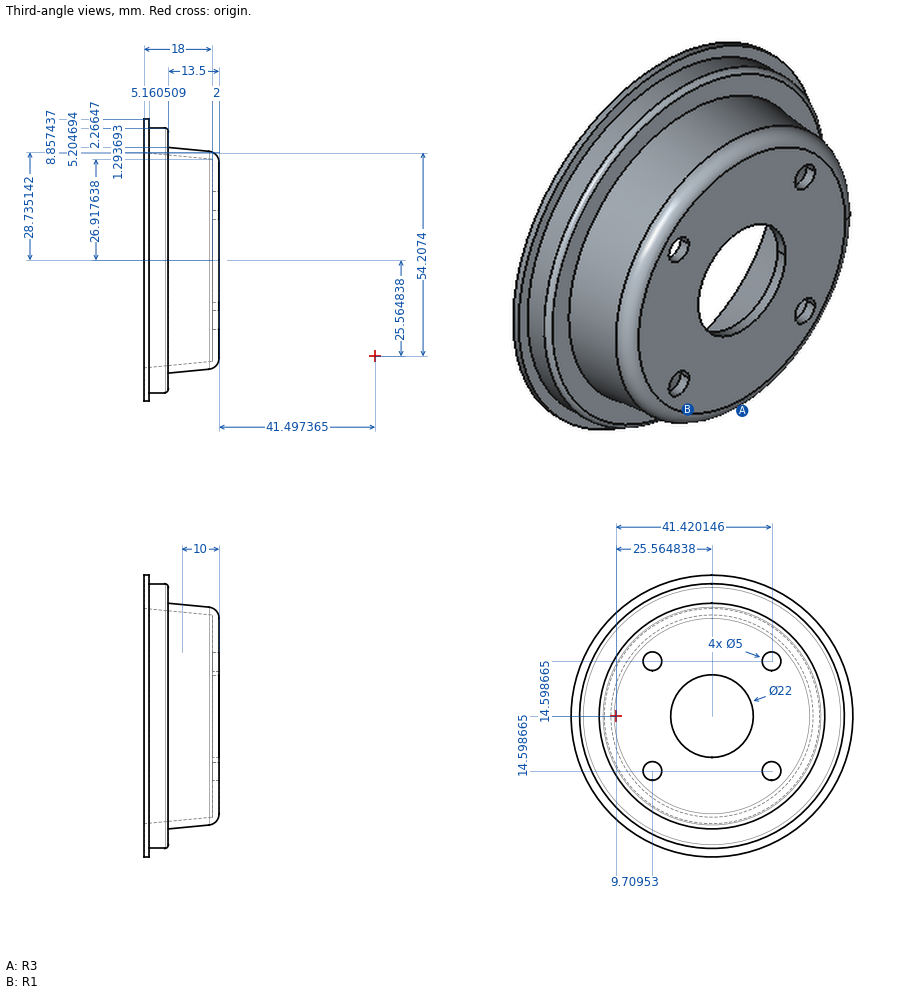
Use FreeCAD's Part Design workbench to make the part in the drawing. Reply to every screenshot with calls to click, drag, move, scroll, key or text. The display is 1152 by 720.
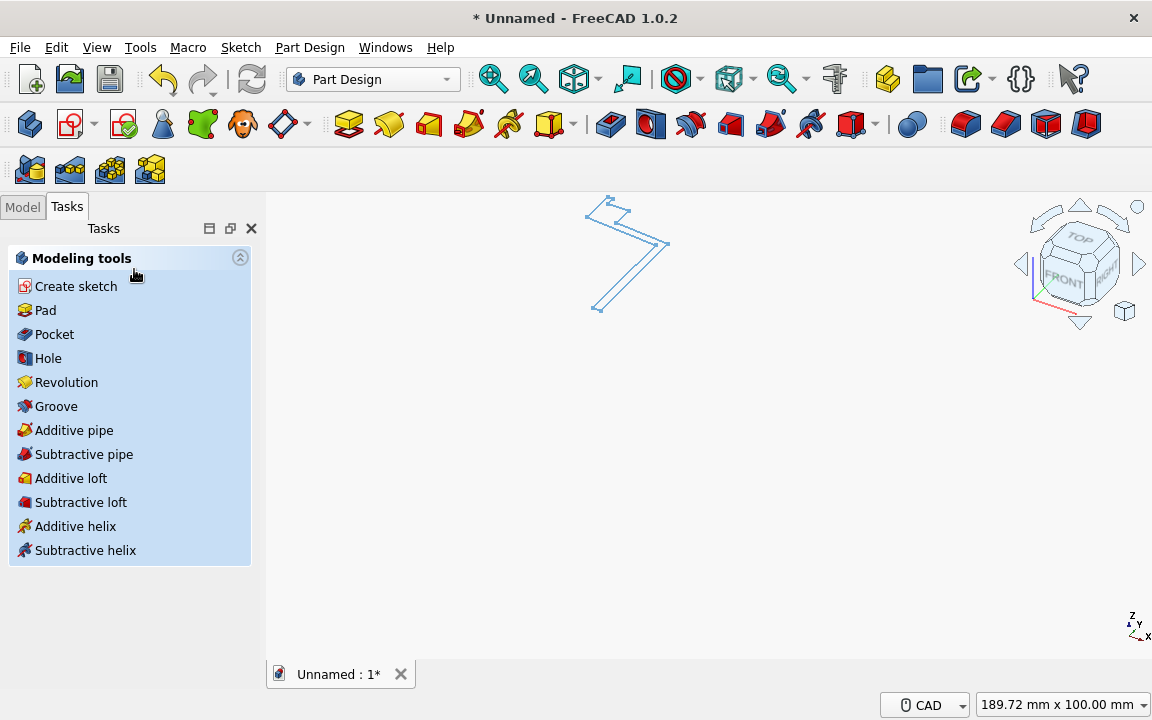
click(390, 124)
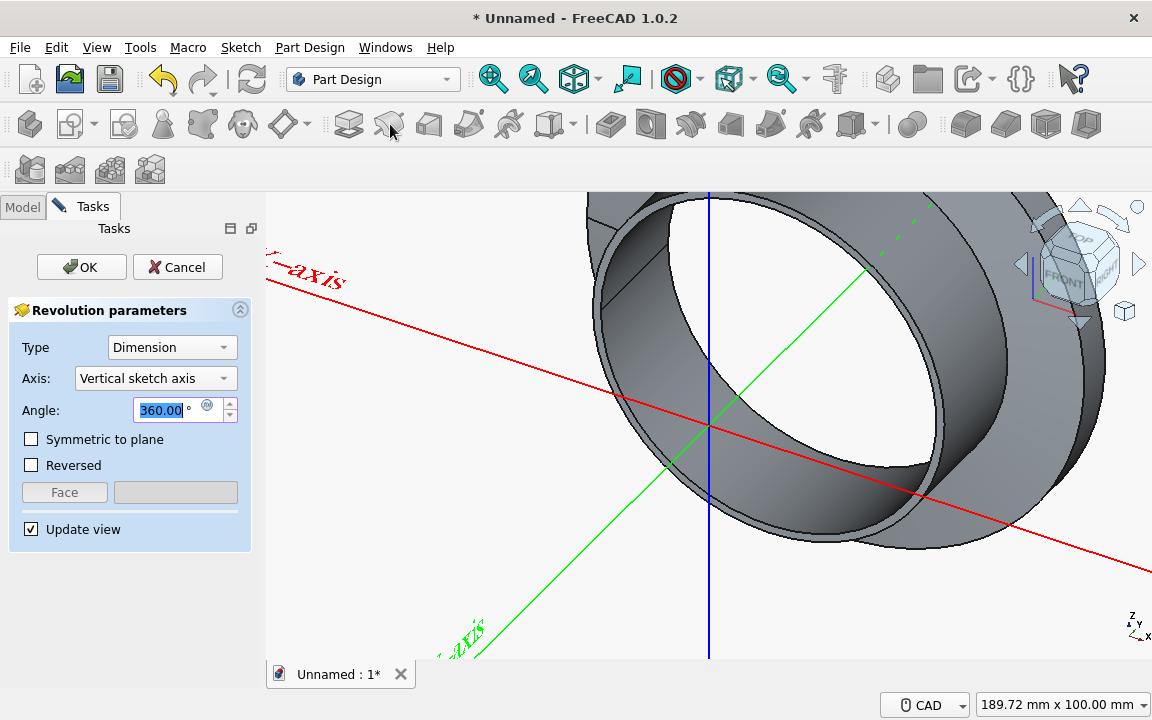
click(156, 378)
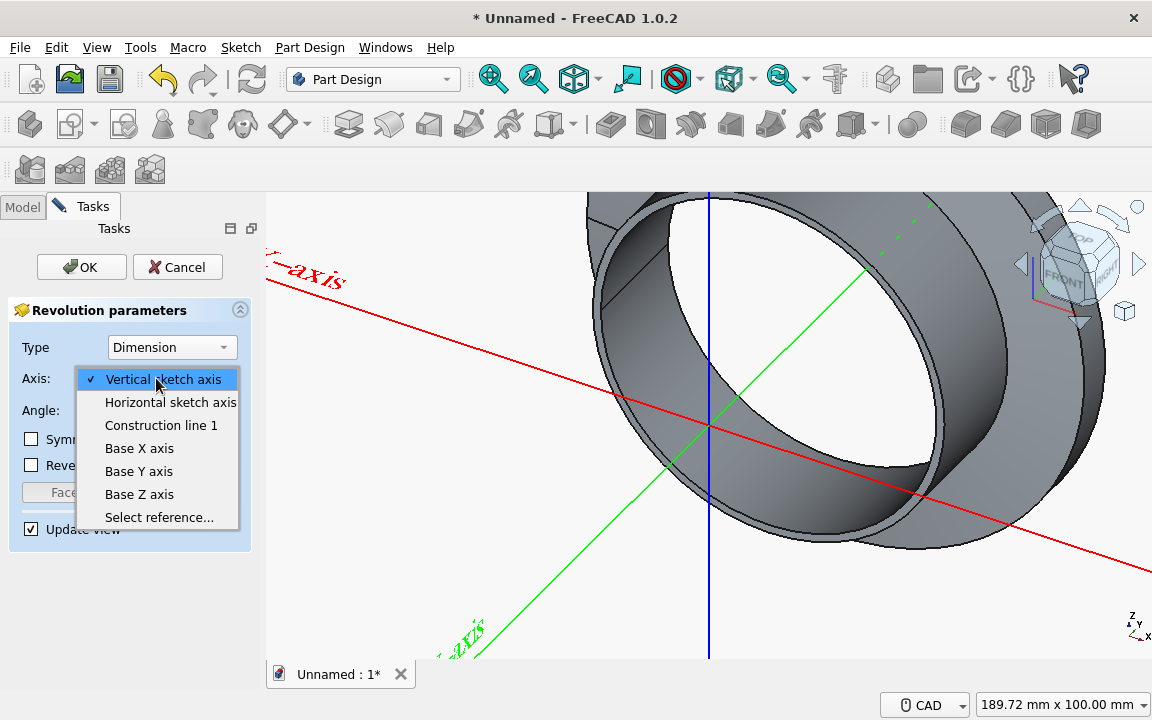
click(156, 426)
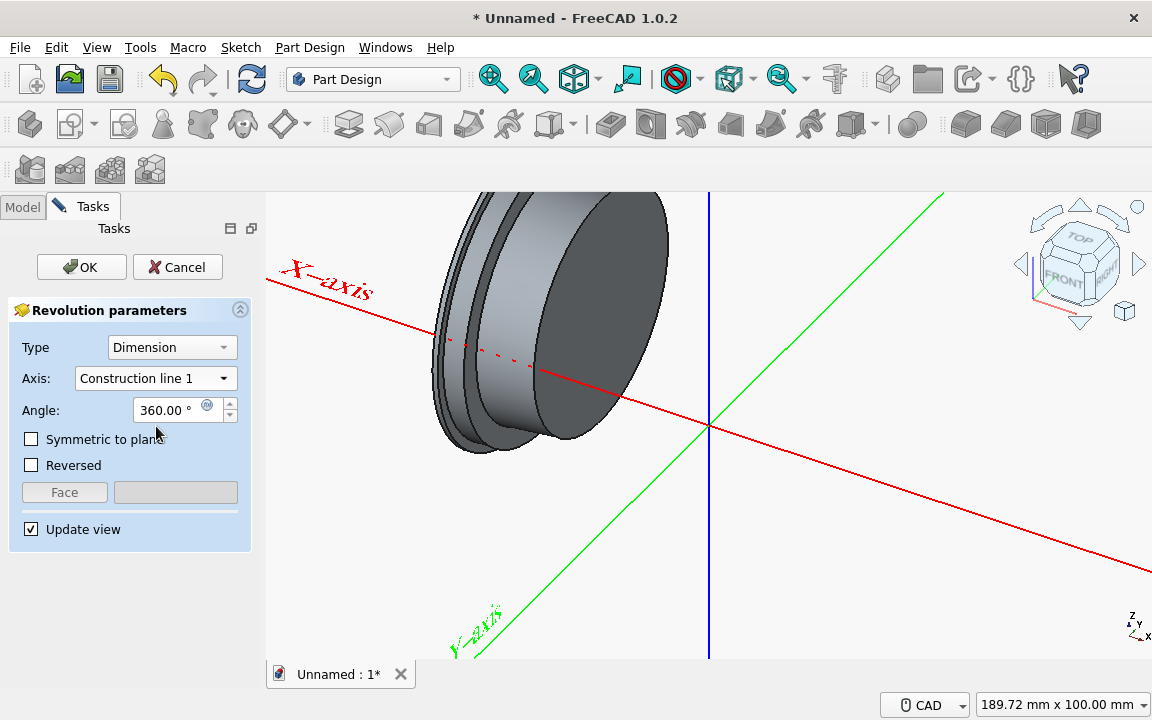
click(82, 267)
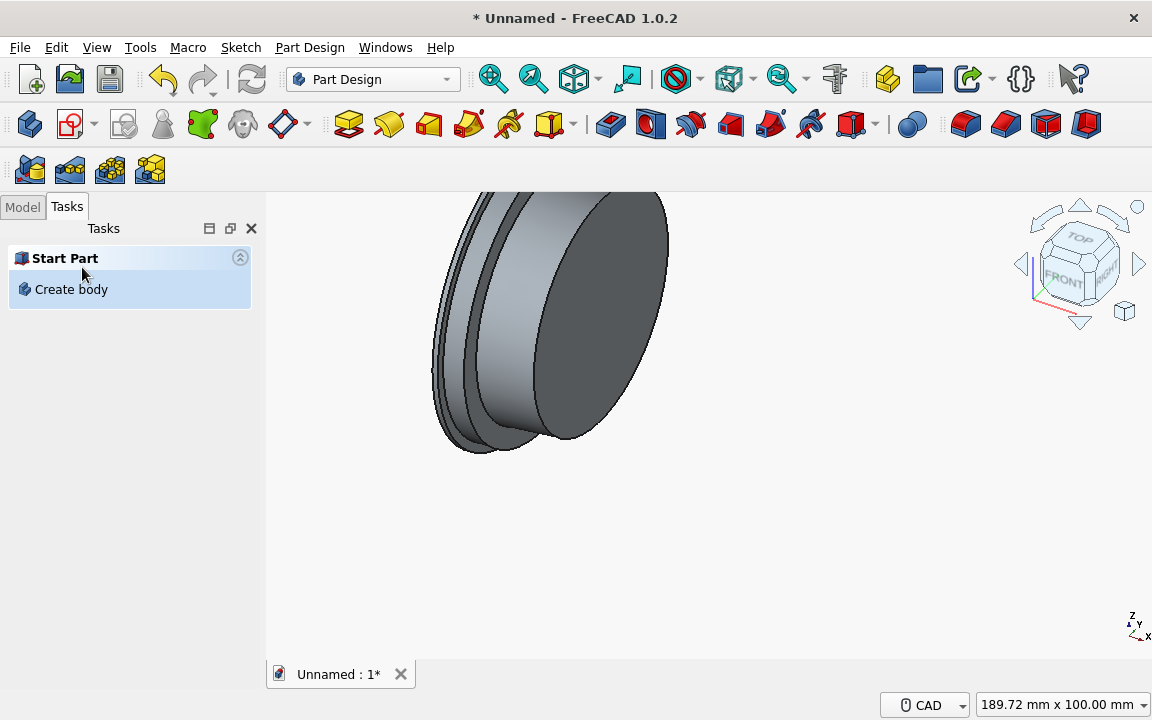
key(v)
key(f)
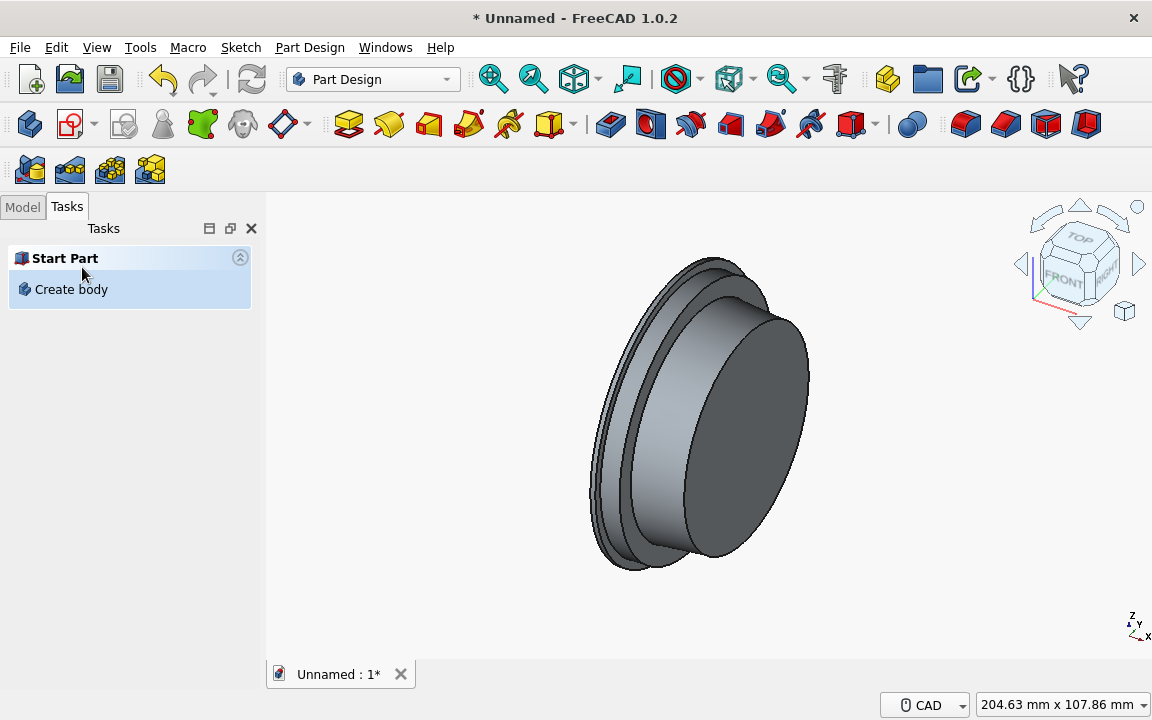
click(746, 437)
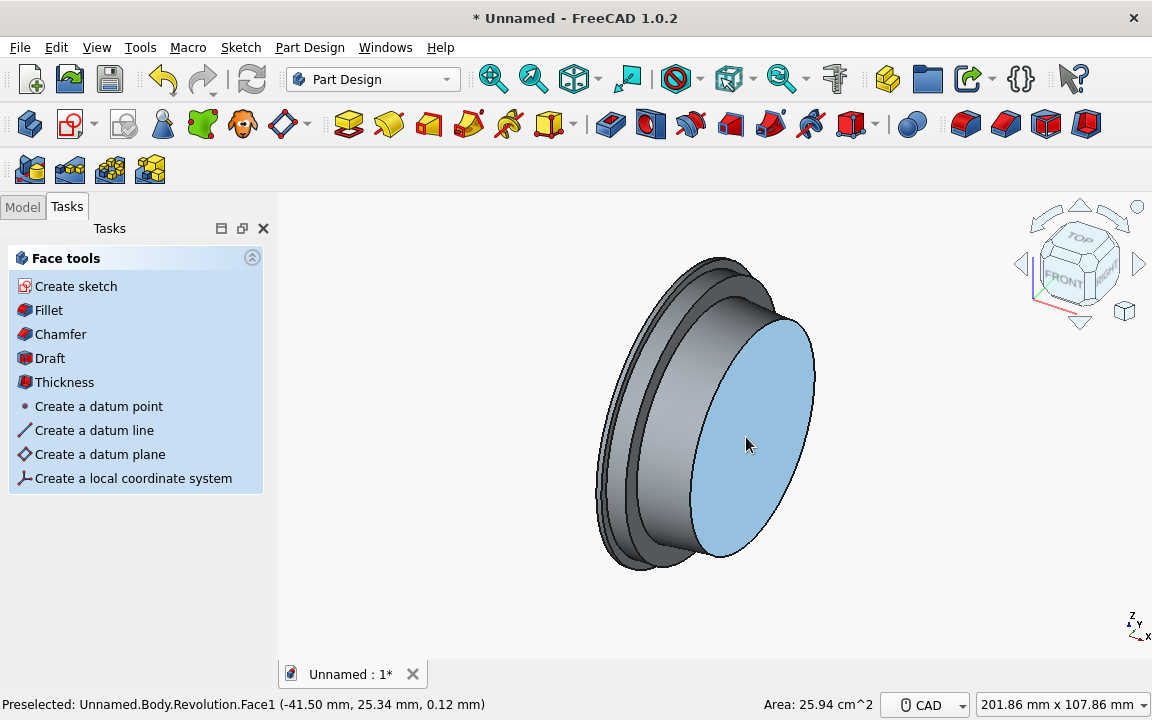
click(70, 124)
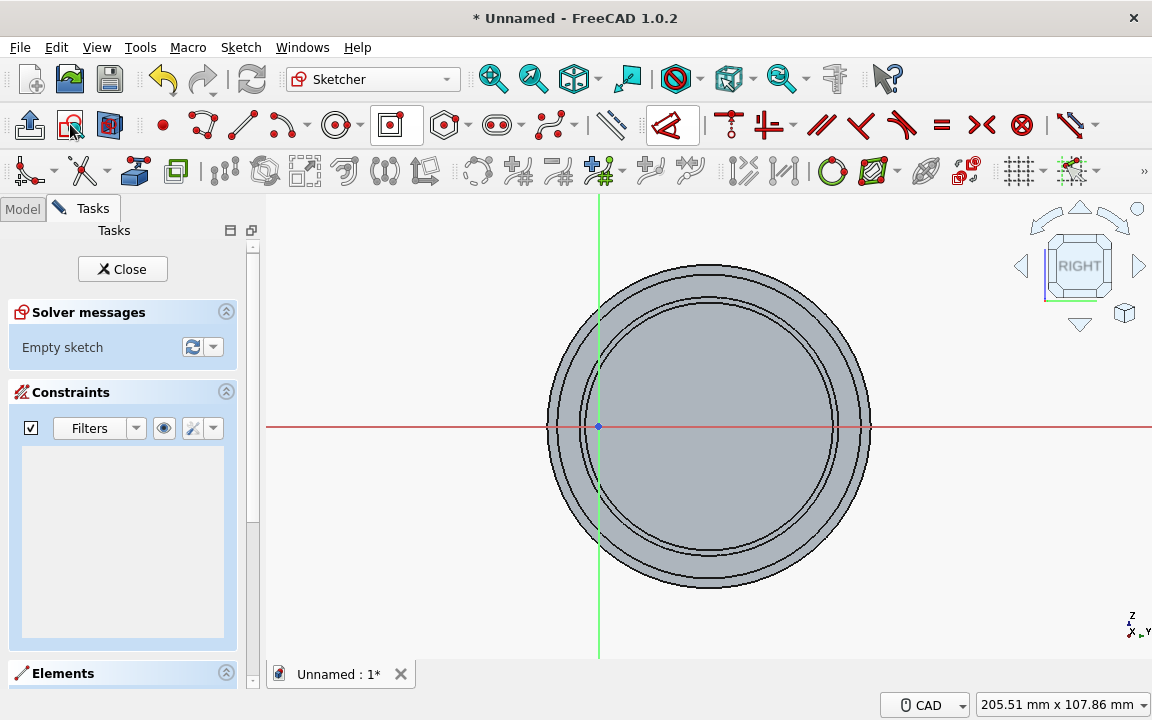
scroll(758, 426, up, 3)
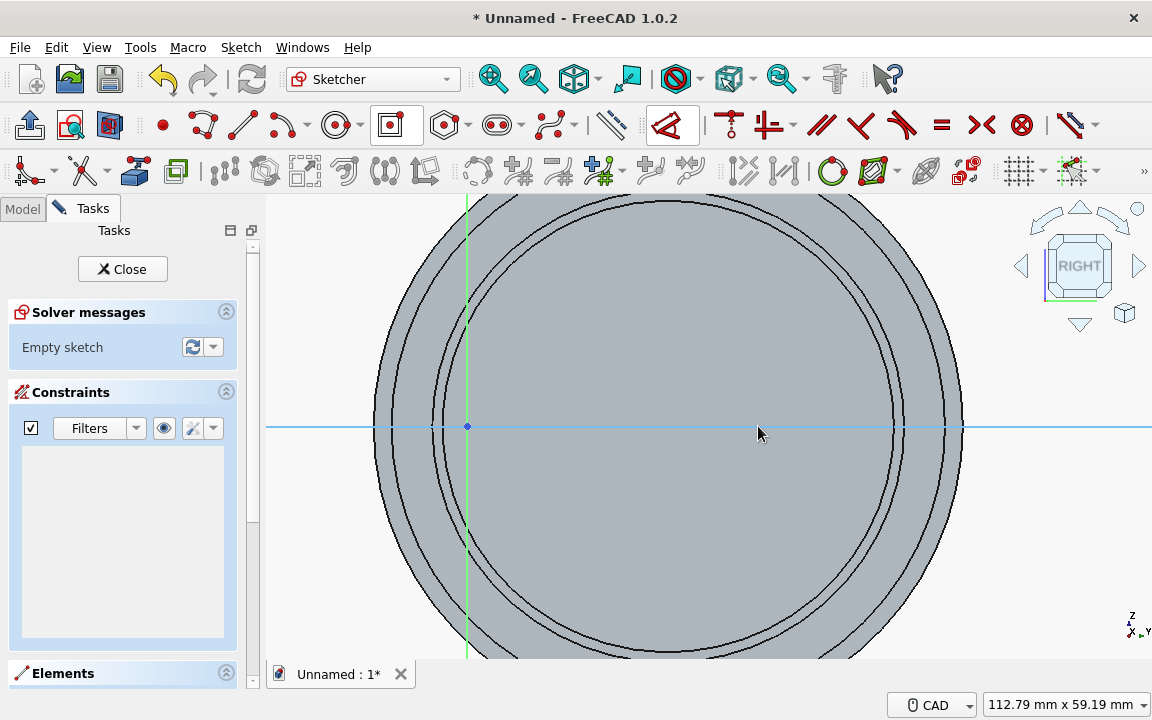
key(g)
key(c)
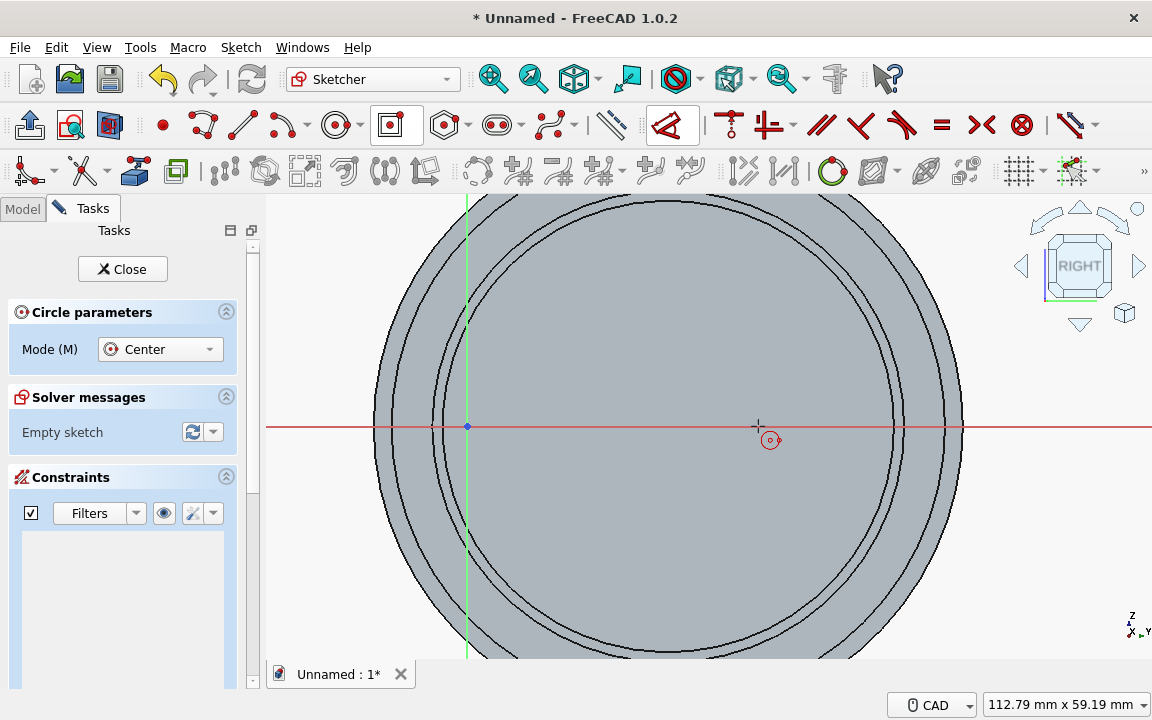
click(668, 426)
move(729, 365)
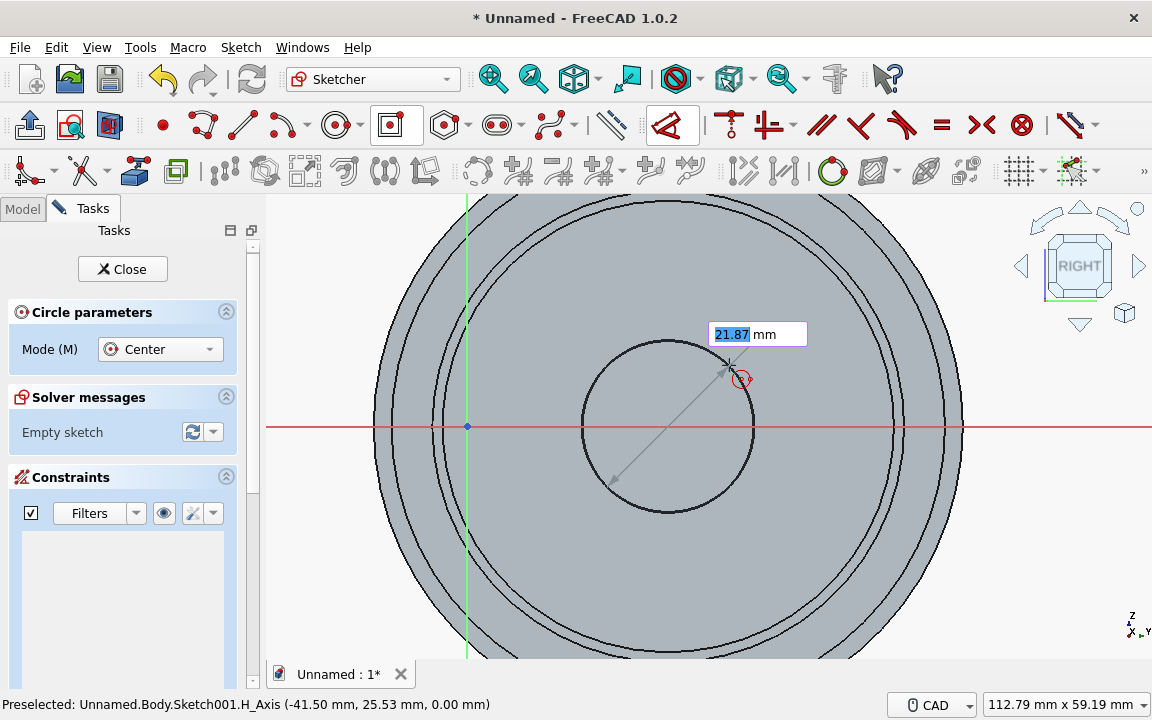
text(22)
key(Return)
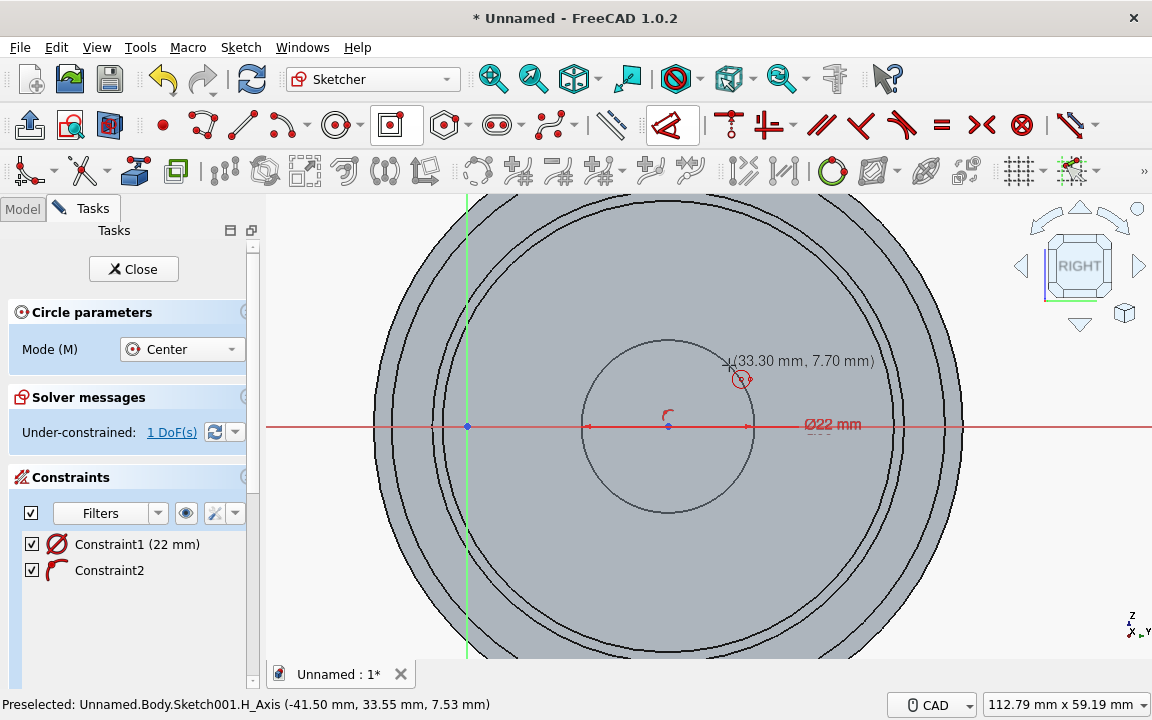
click(793, 312)
move(807, 298)